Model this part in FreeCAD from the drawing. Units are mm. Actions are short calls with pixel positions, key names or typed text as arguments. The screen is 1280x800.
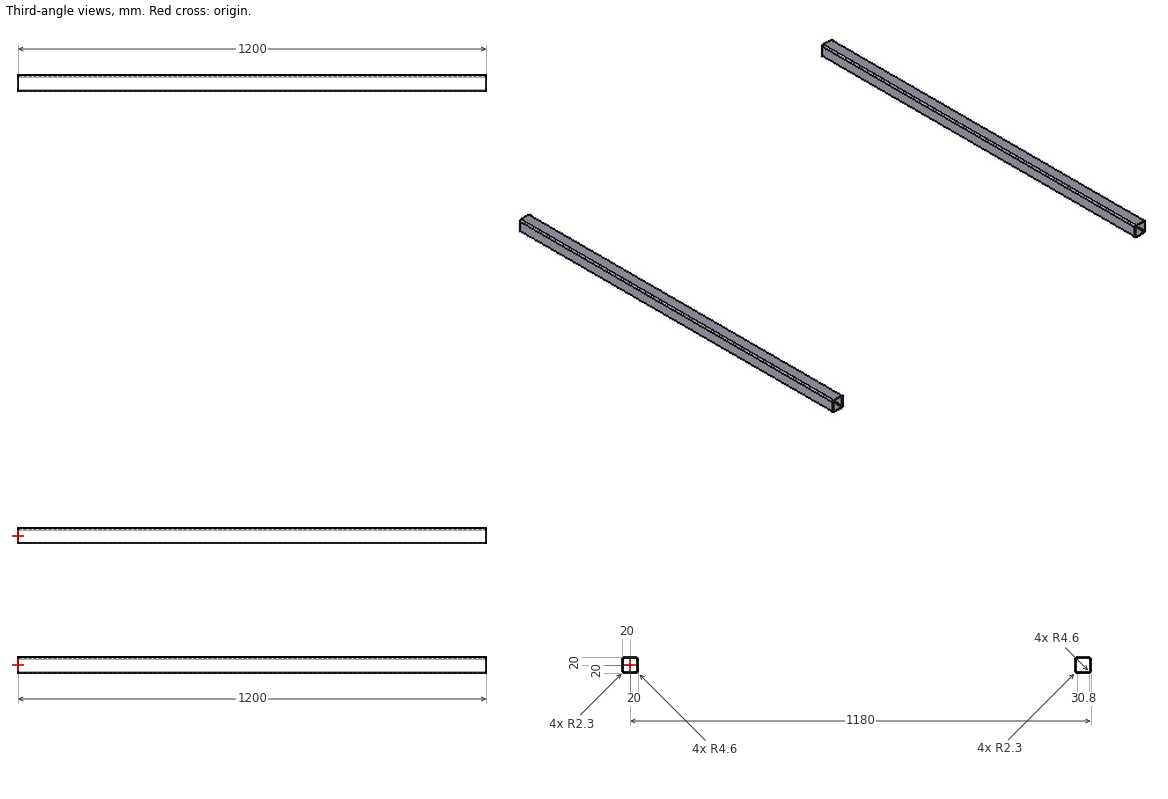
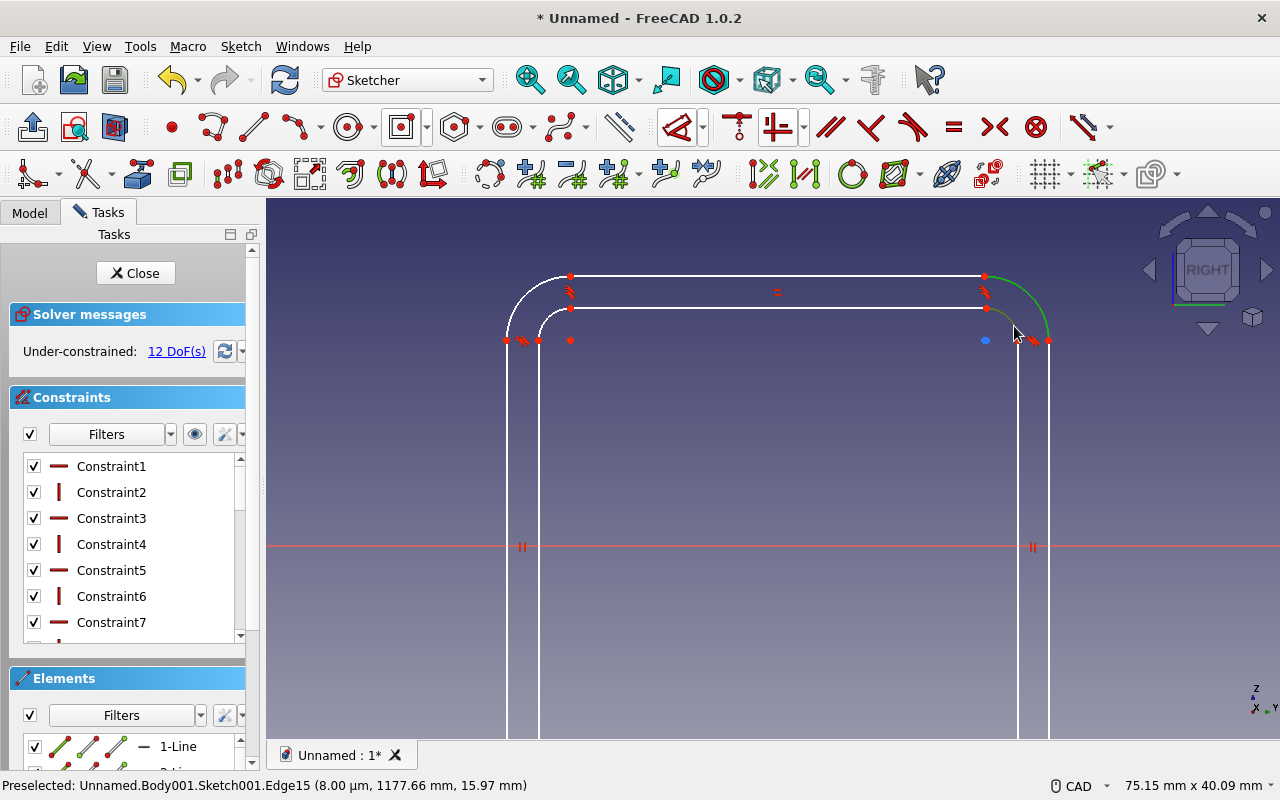
key(c)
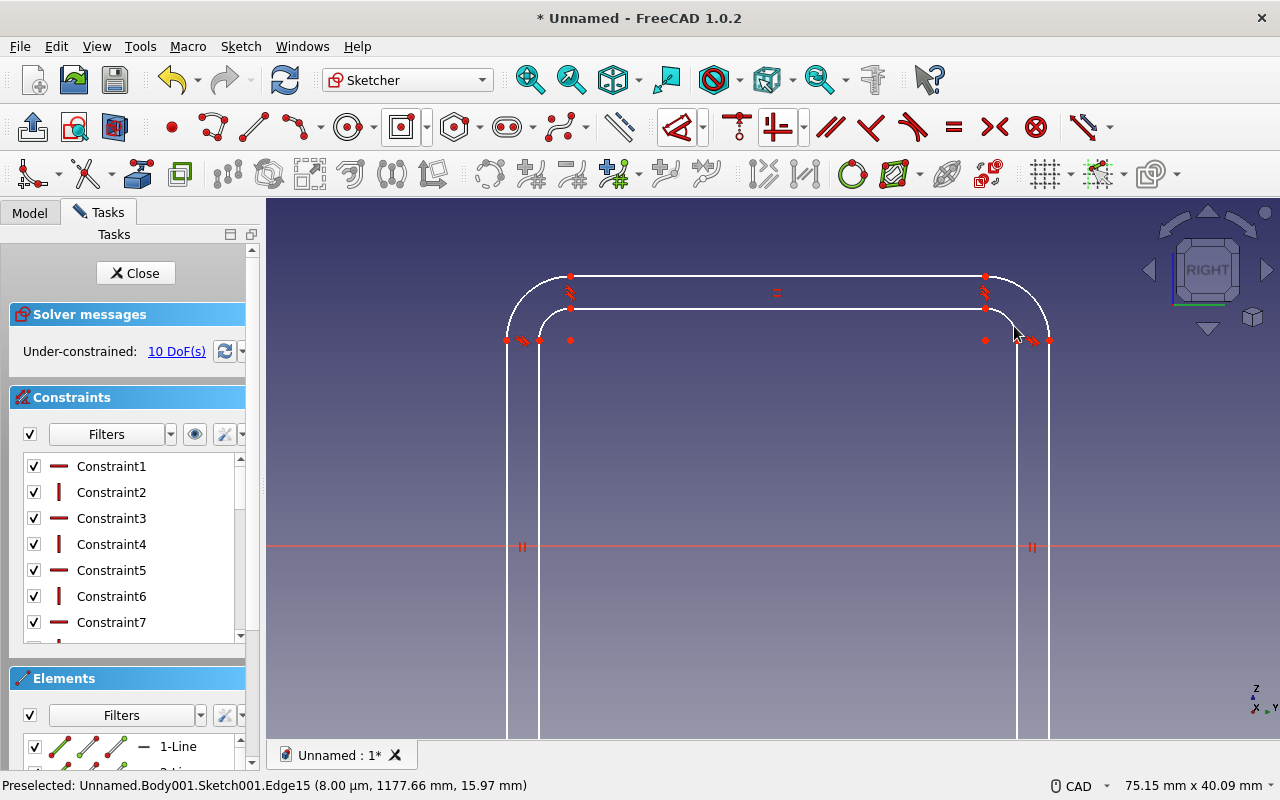
scroll(555, 311, down, 2)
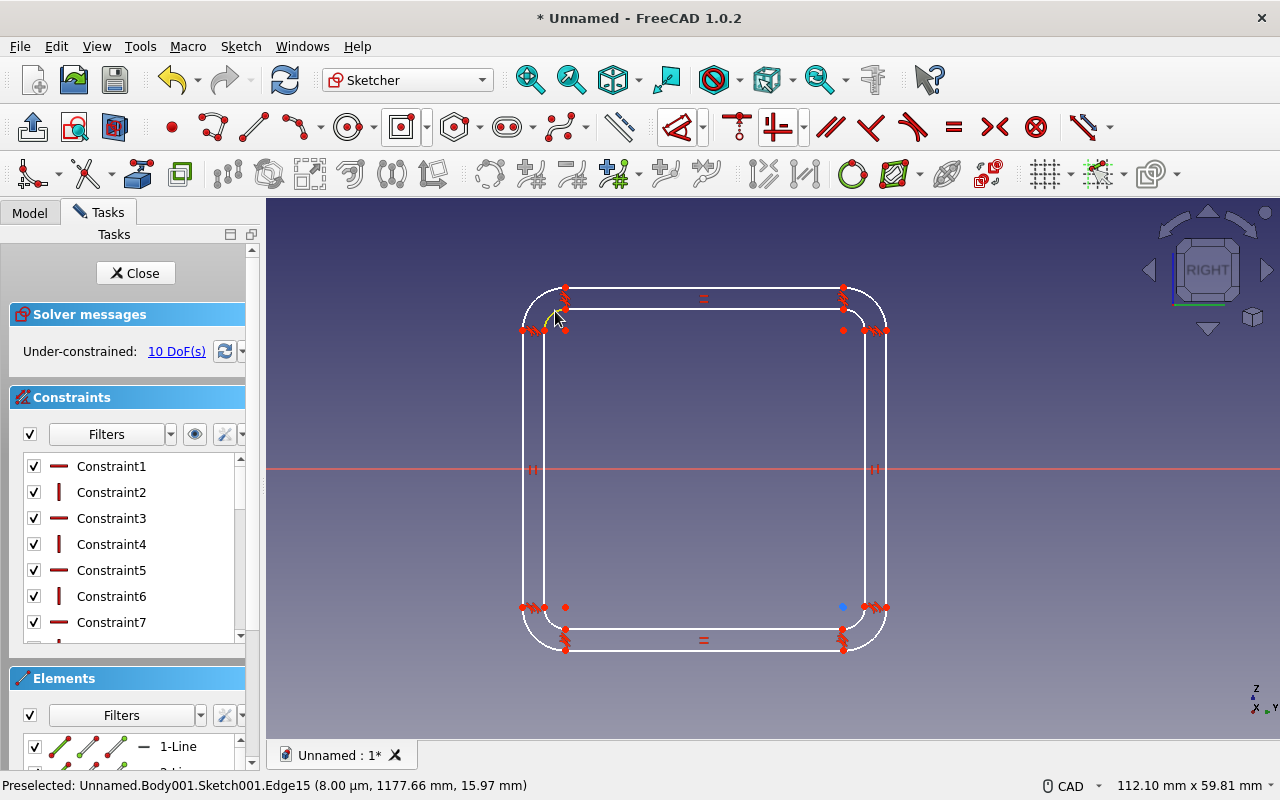
click(863, 646)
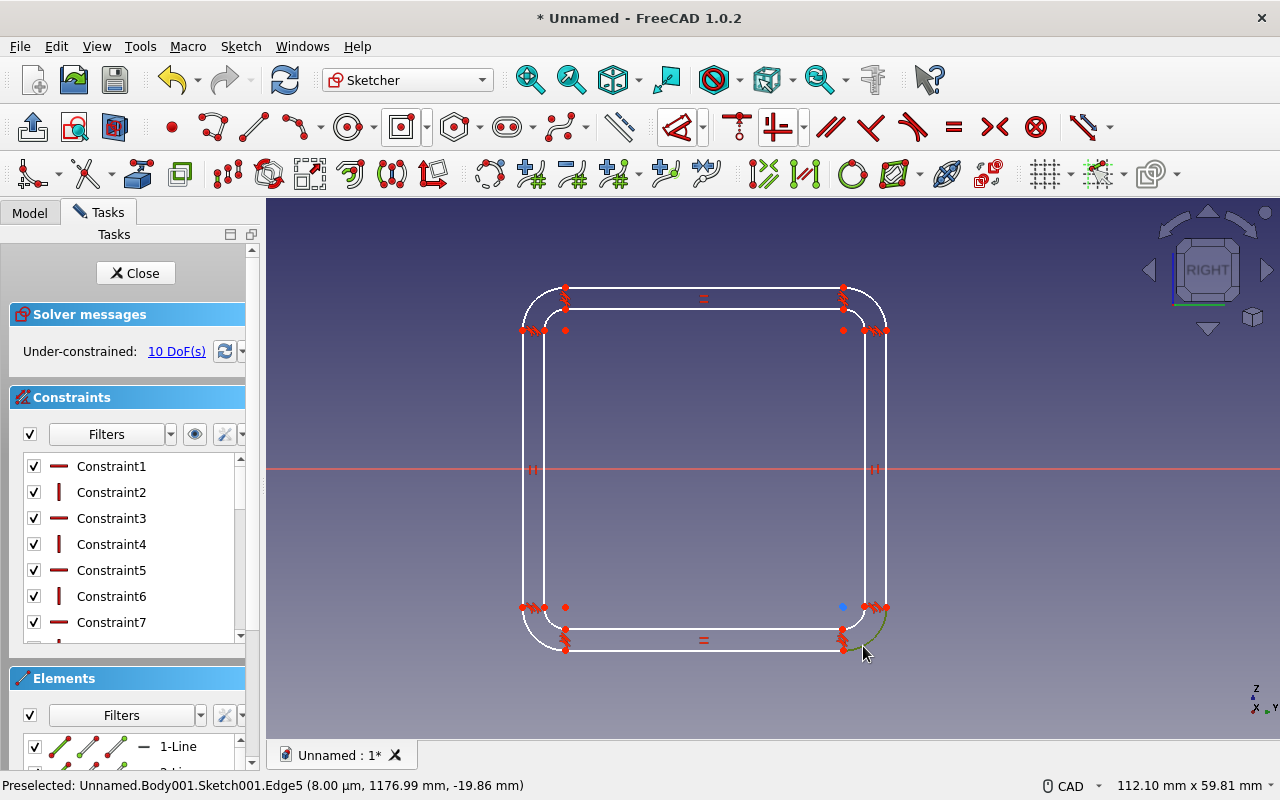
click(882, 311)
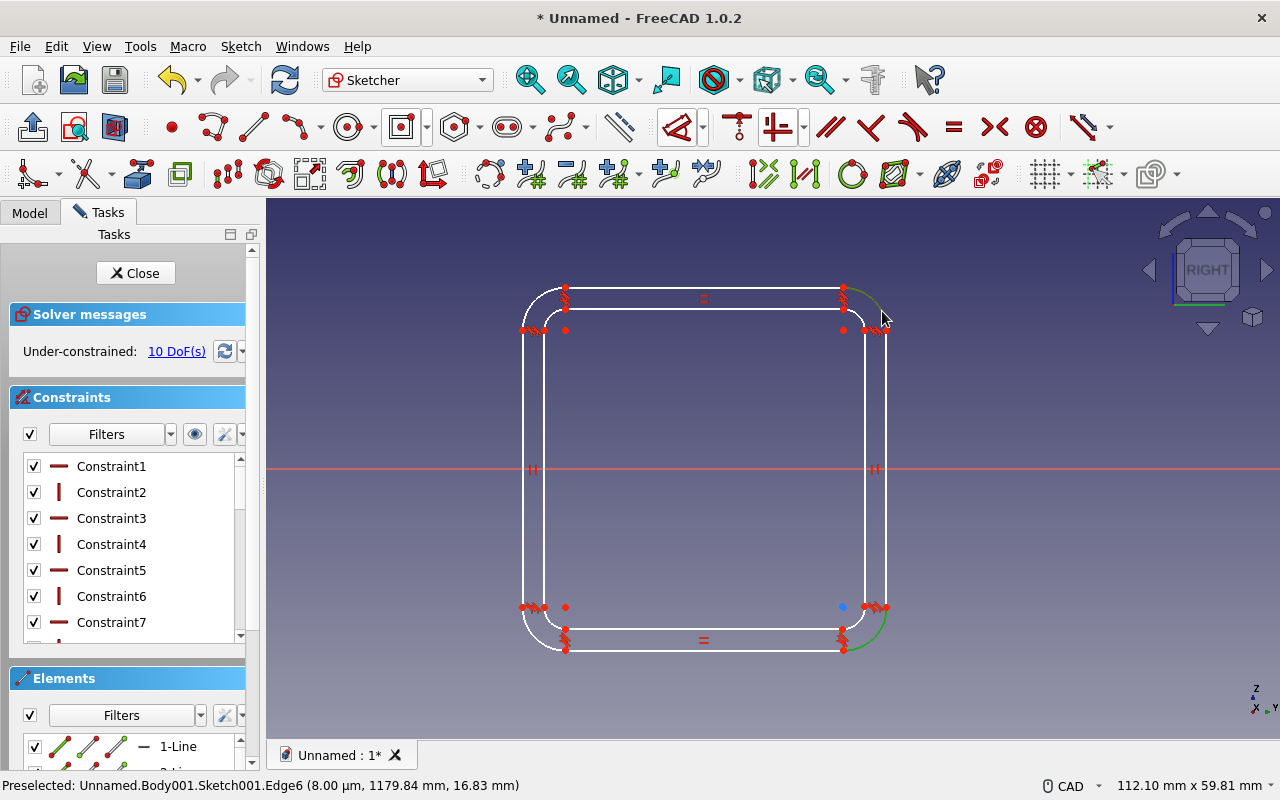
click(546, 293)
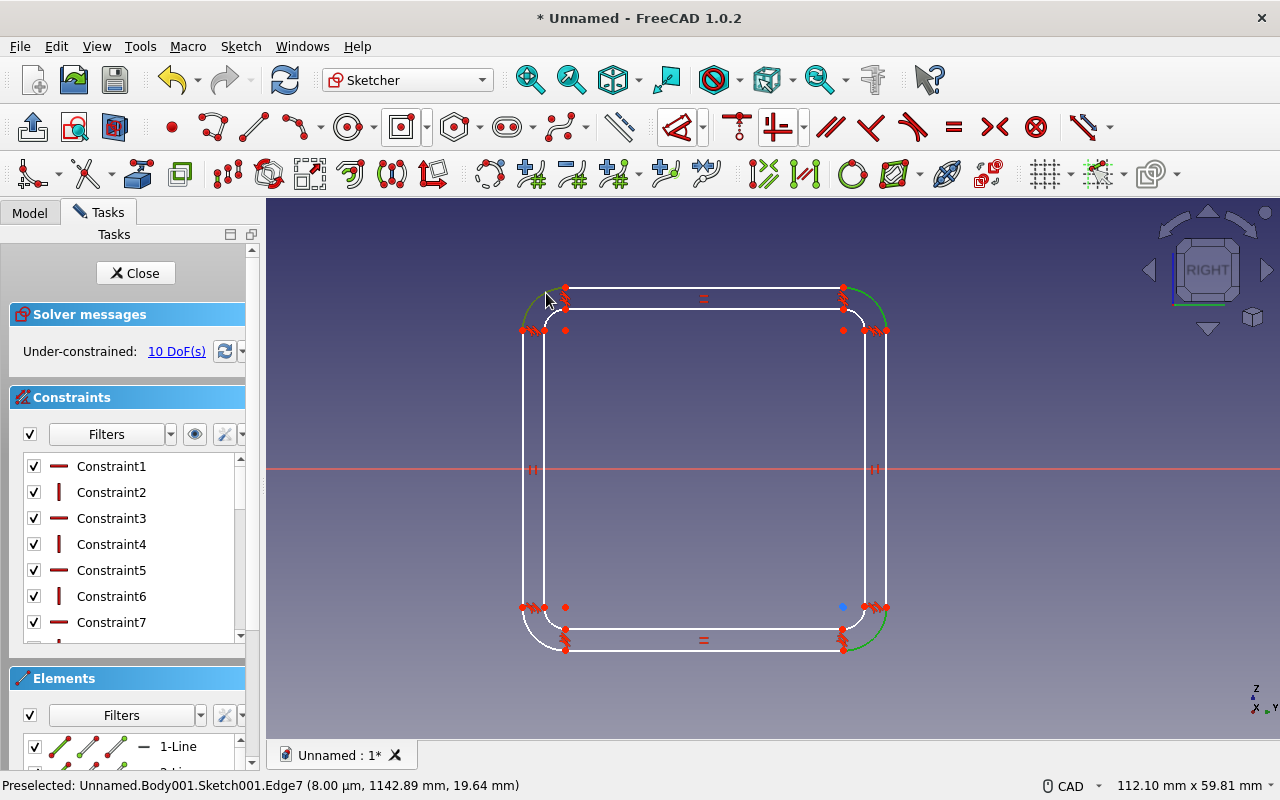
click(528, 627)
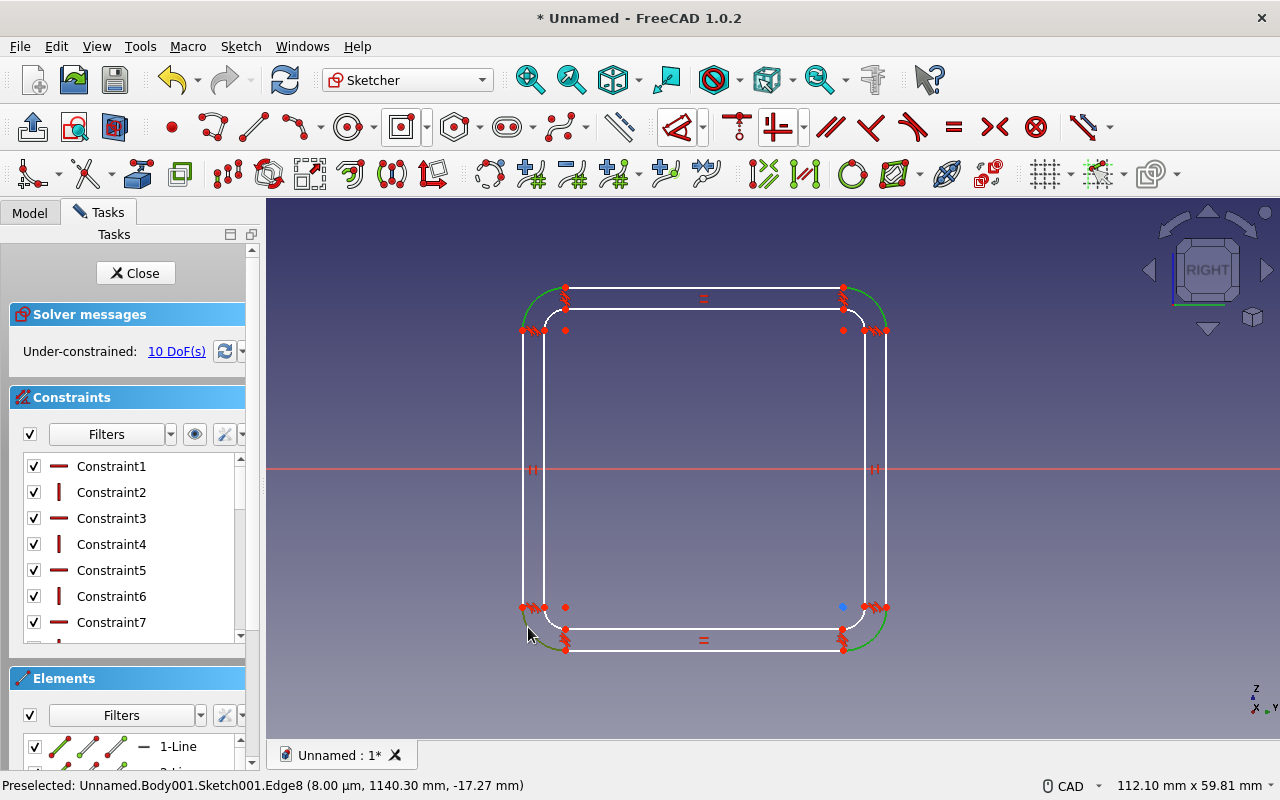
key(e)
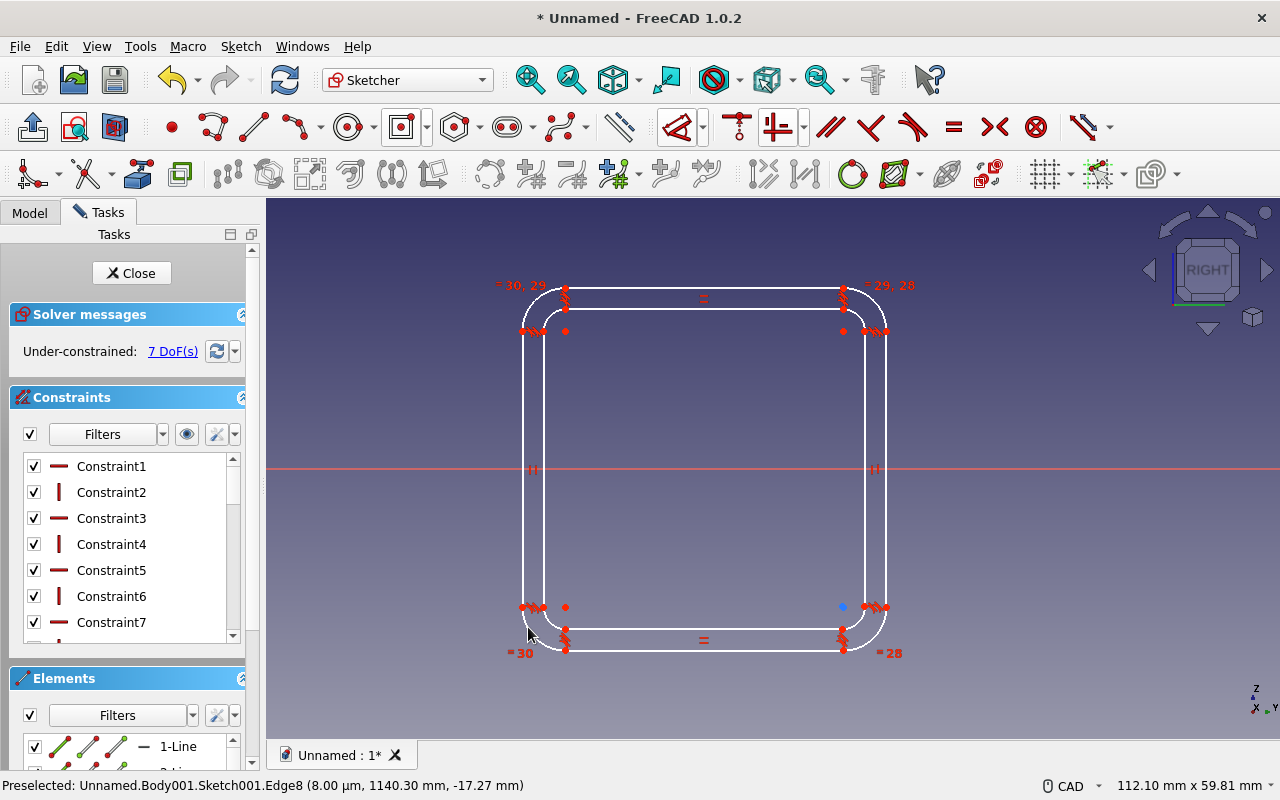
scroll(546, 617, up, 2)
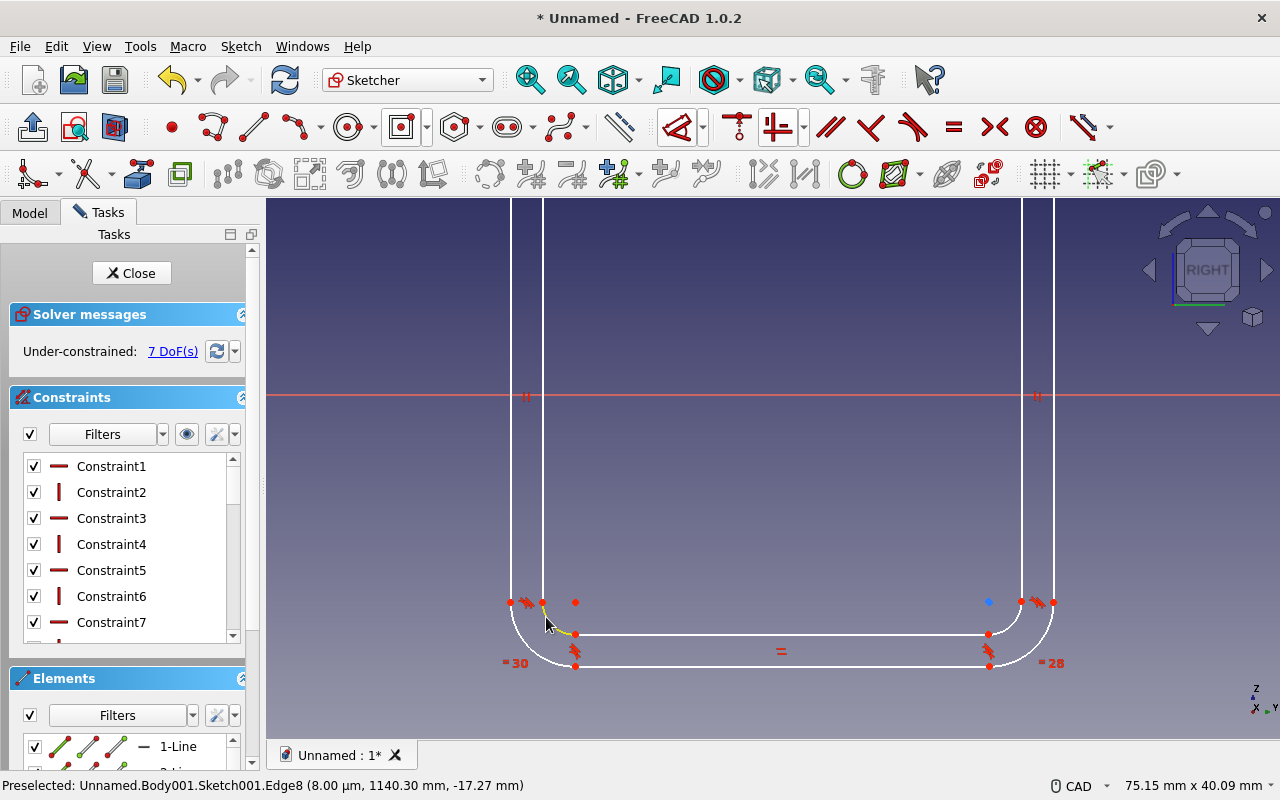
click(546, 617)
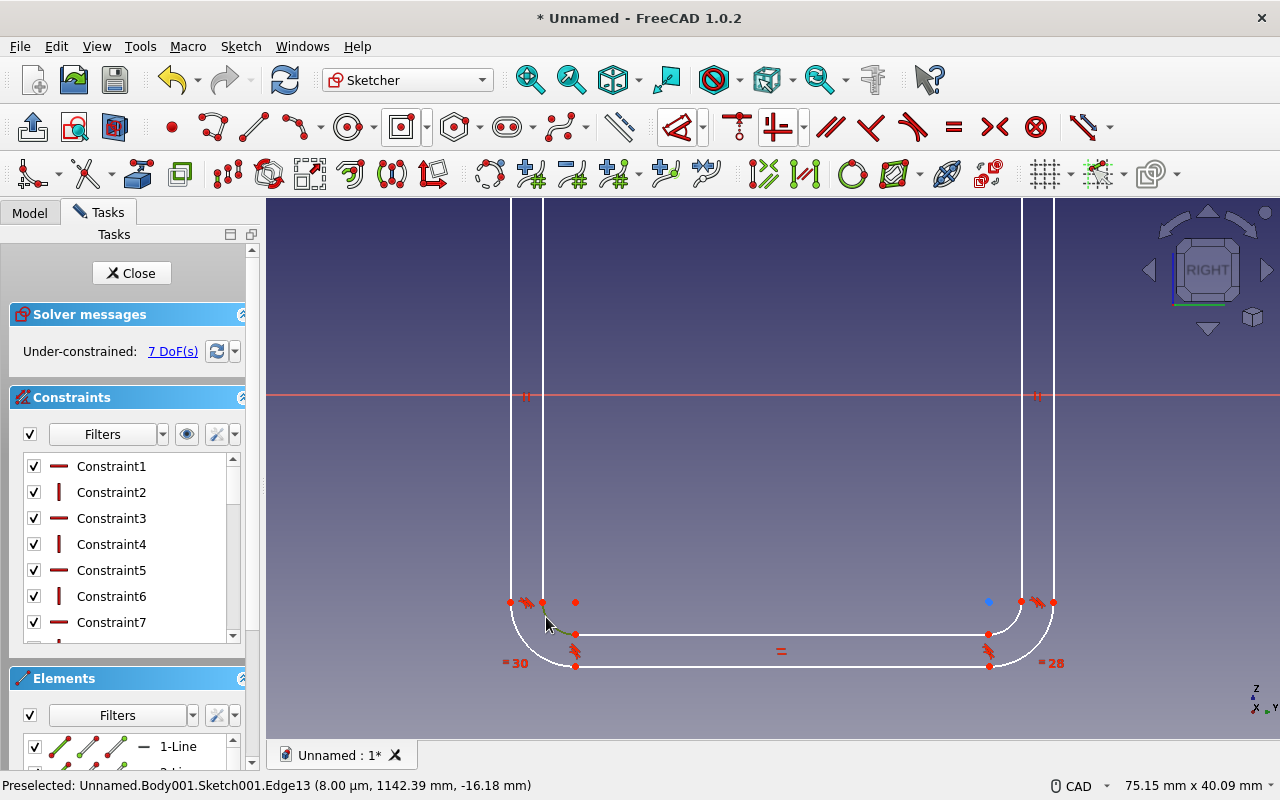
click(1003, 631)